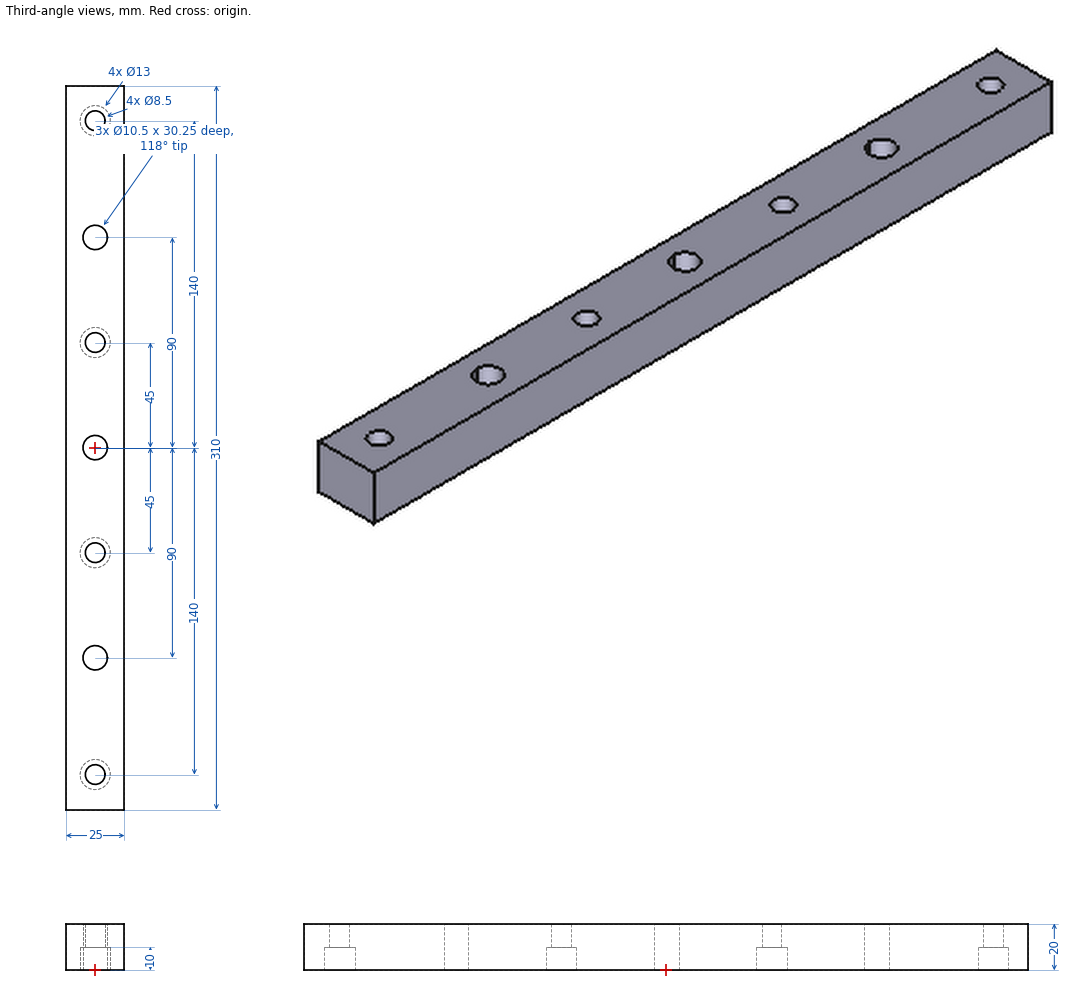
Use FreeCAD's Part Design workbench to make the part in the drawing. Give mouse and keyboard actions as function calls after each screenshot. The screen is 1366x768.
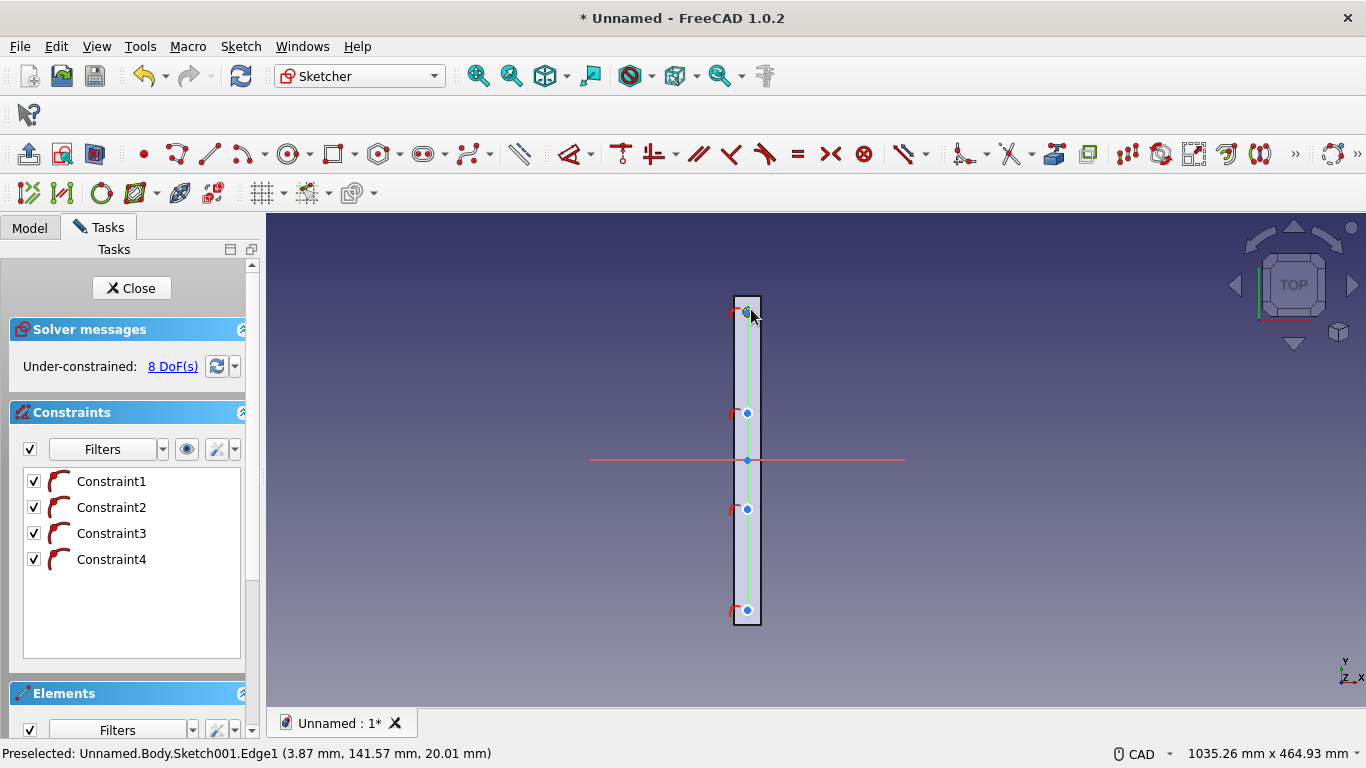
scroll(751, 410, up, 8)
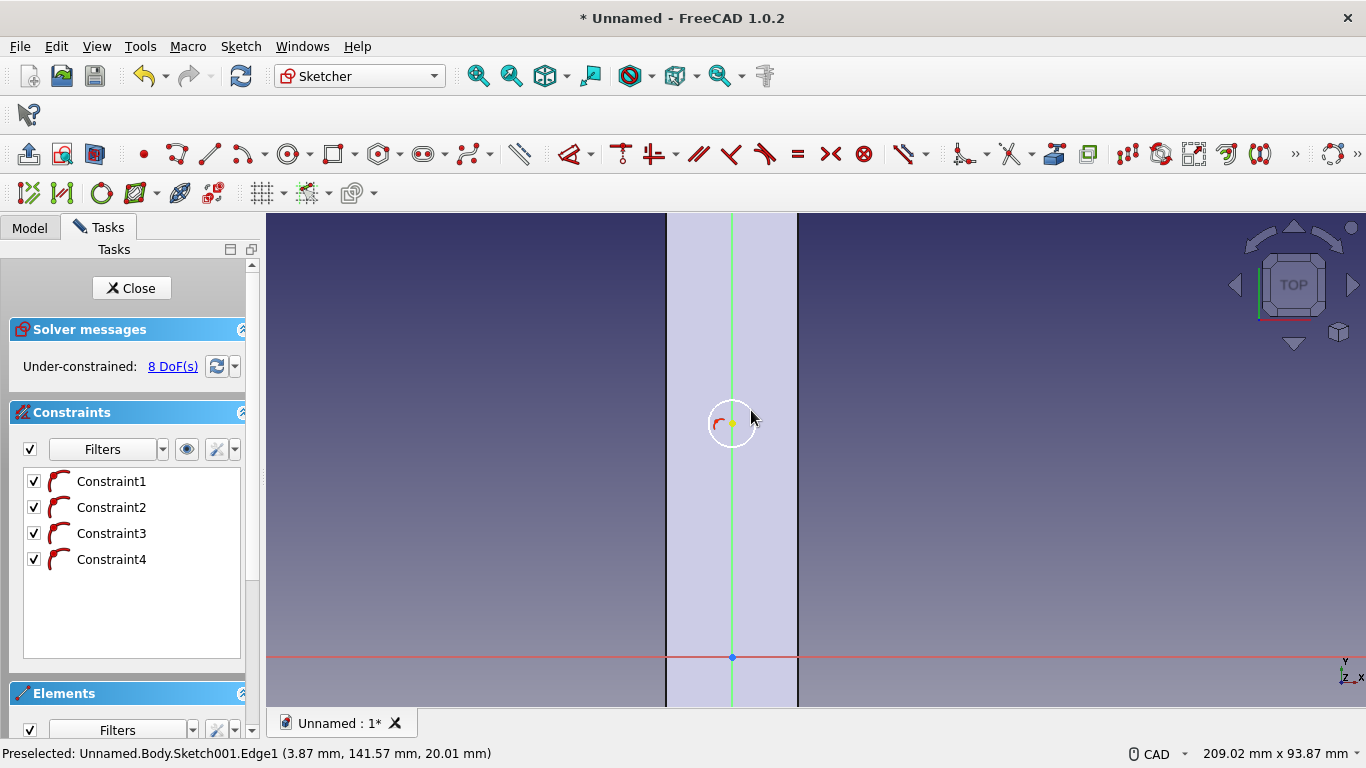
click(749, 407)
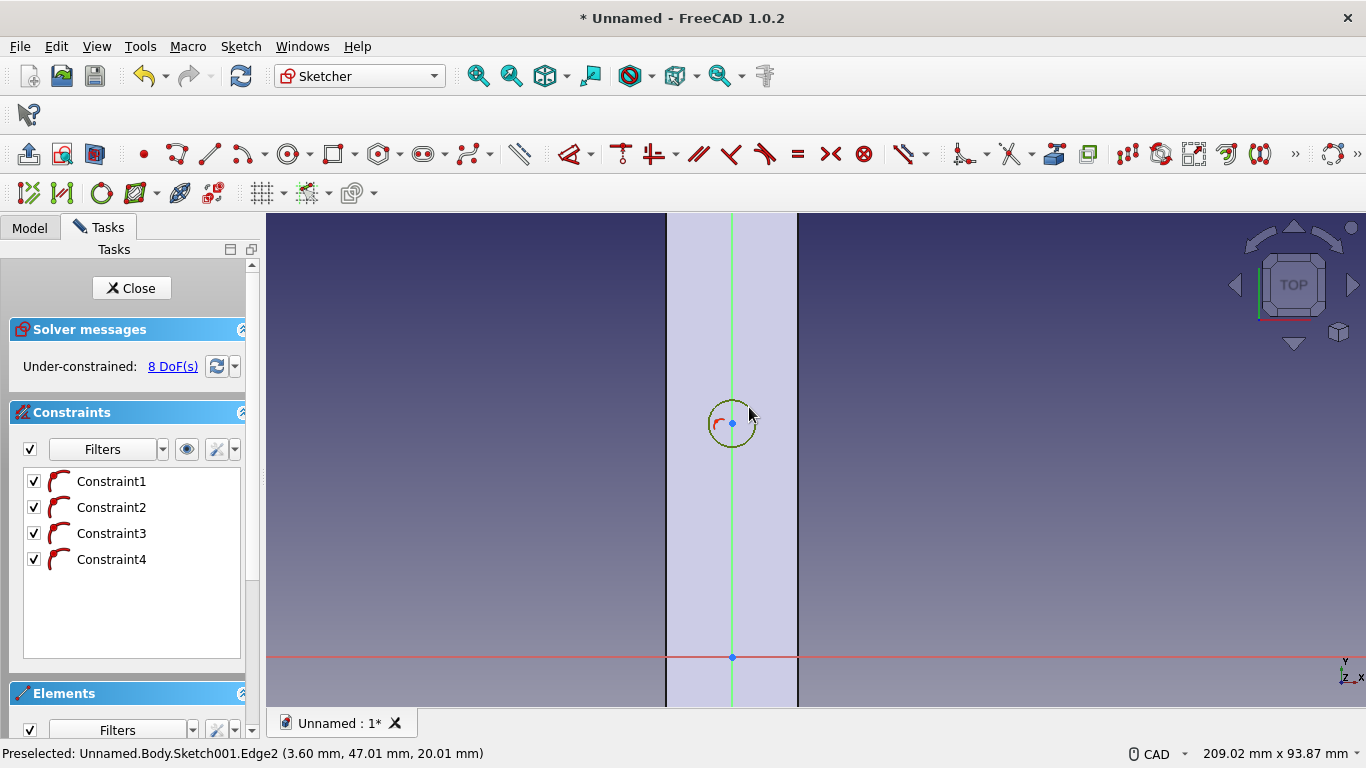
scroll(751, 410, down, 8)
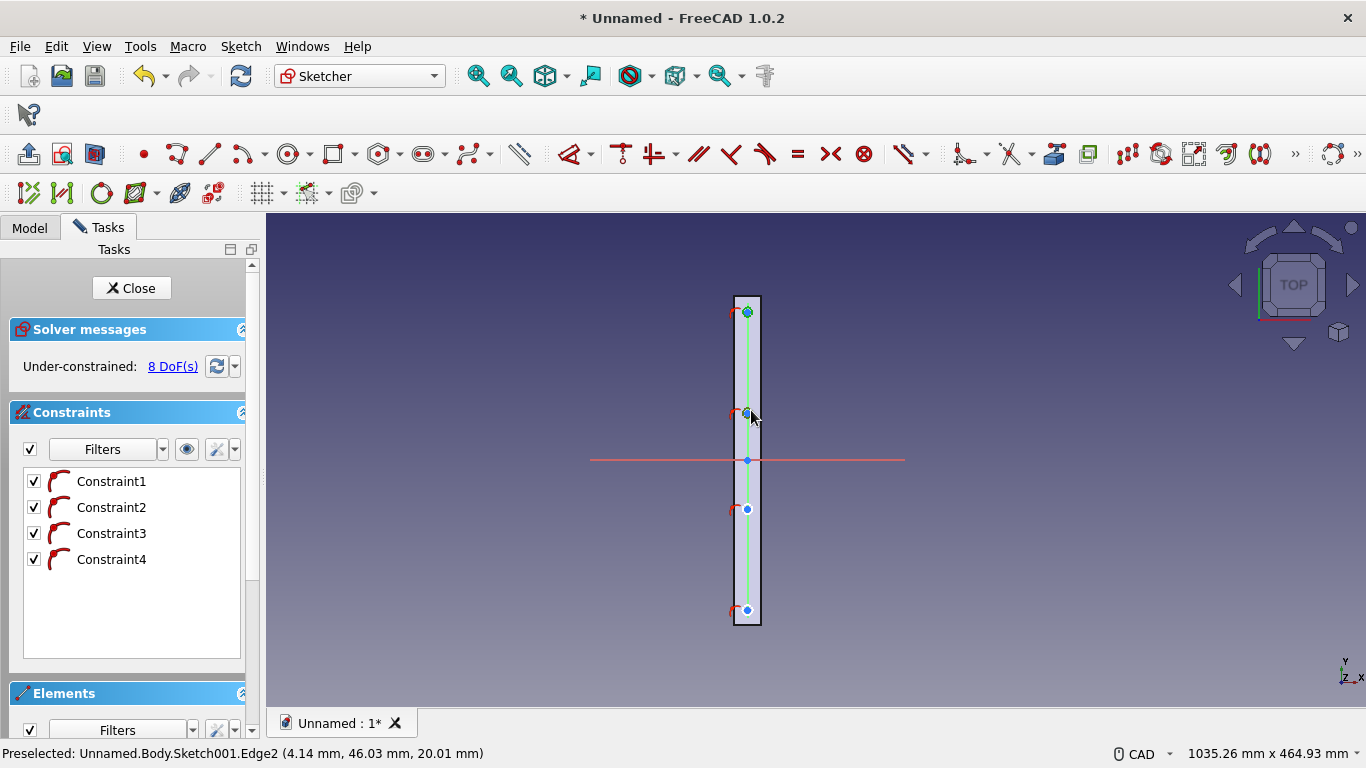
scroll(751, 506, up, 7)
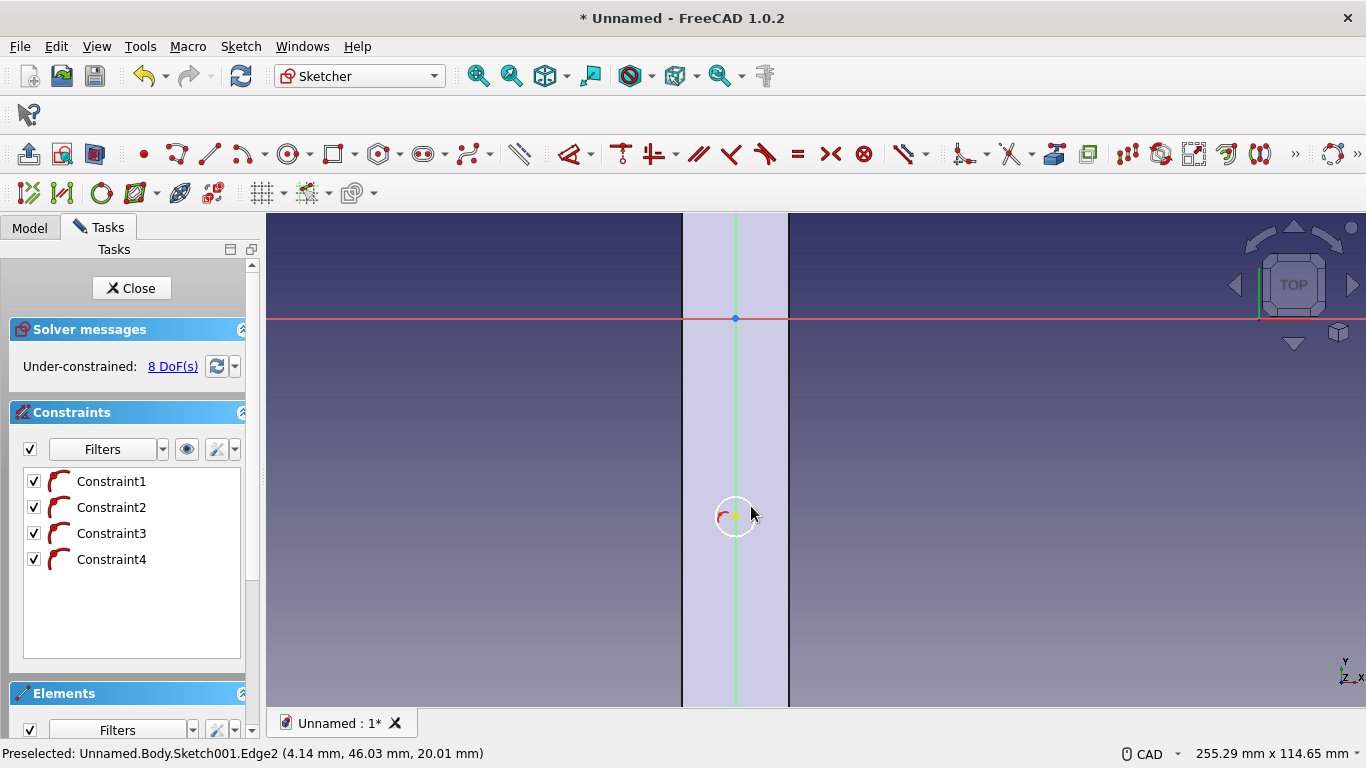
click(750, 503)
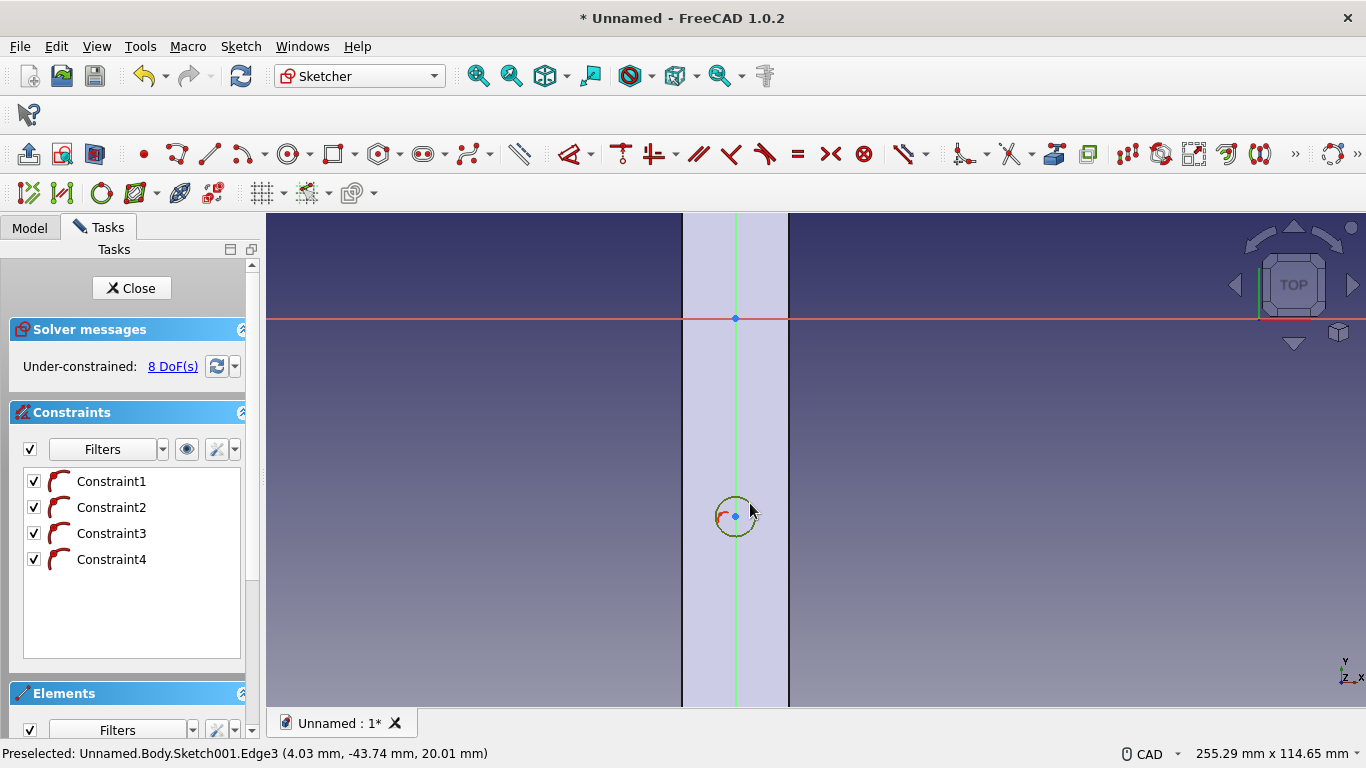
scroll(751, 506, down, 7)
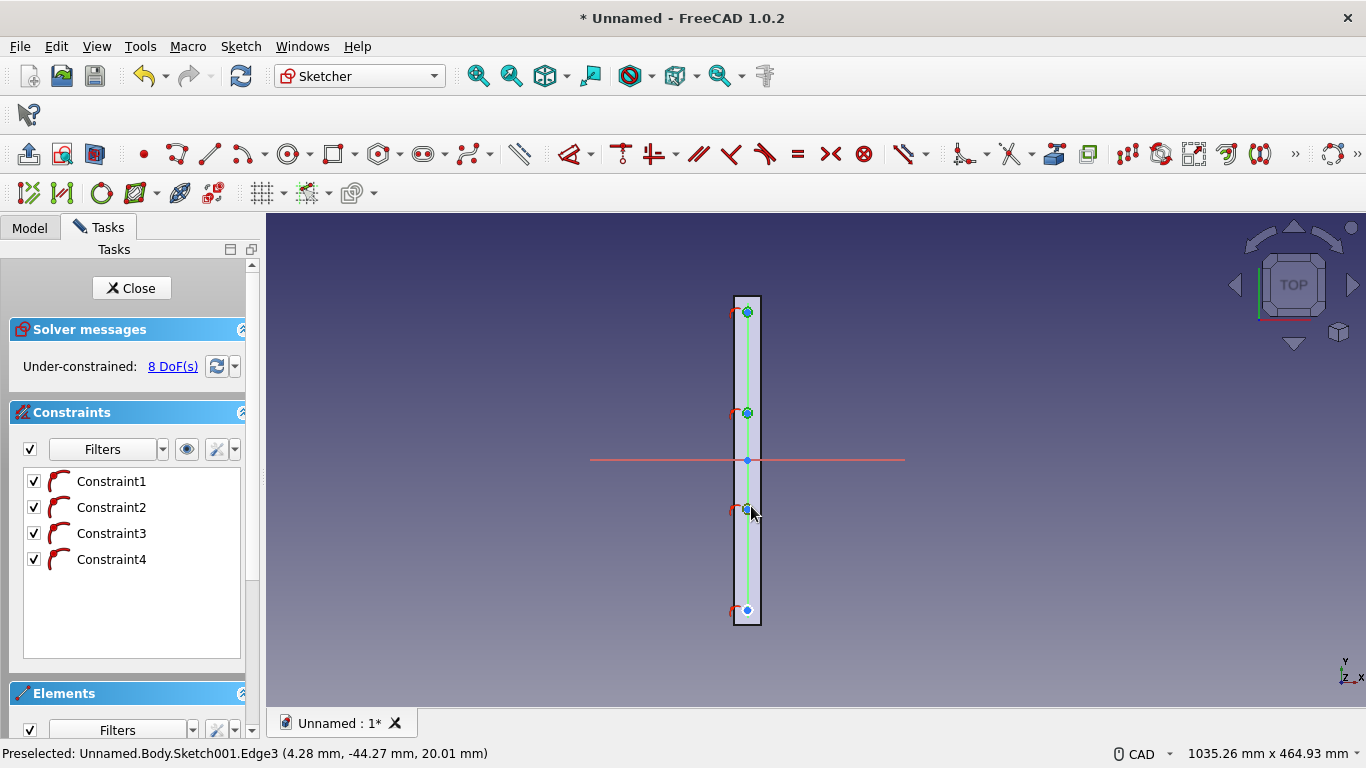
scroll(751, 607, up, 7)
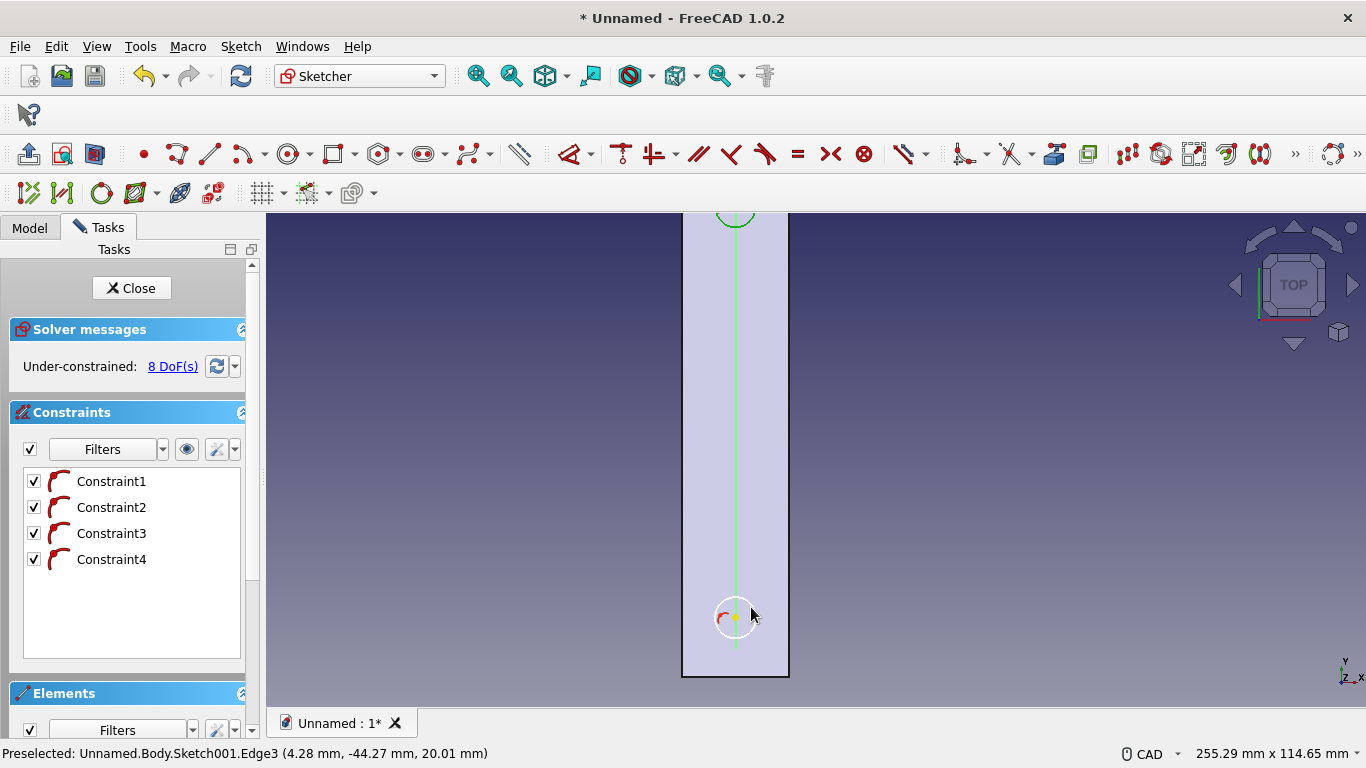
click(750, 603)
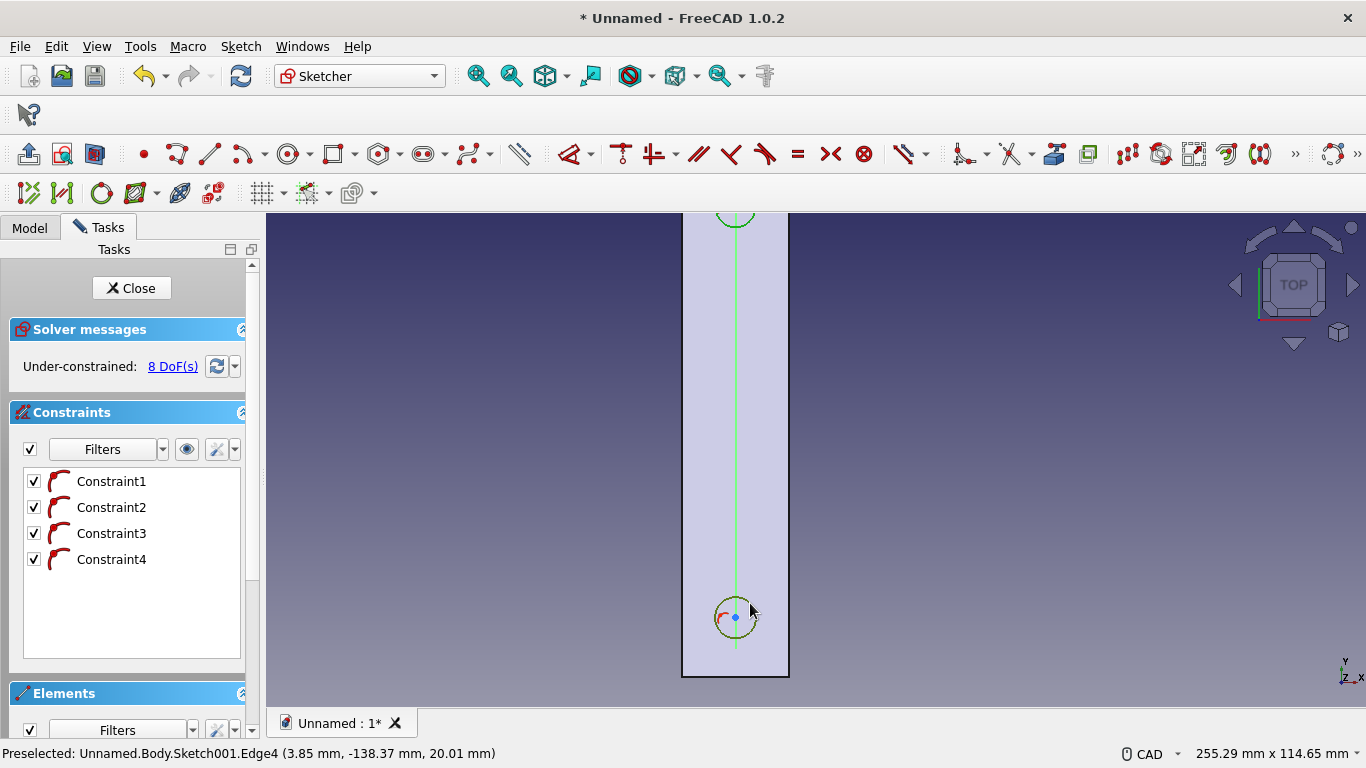
click(798, 154)